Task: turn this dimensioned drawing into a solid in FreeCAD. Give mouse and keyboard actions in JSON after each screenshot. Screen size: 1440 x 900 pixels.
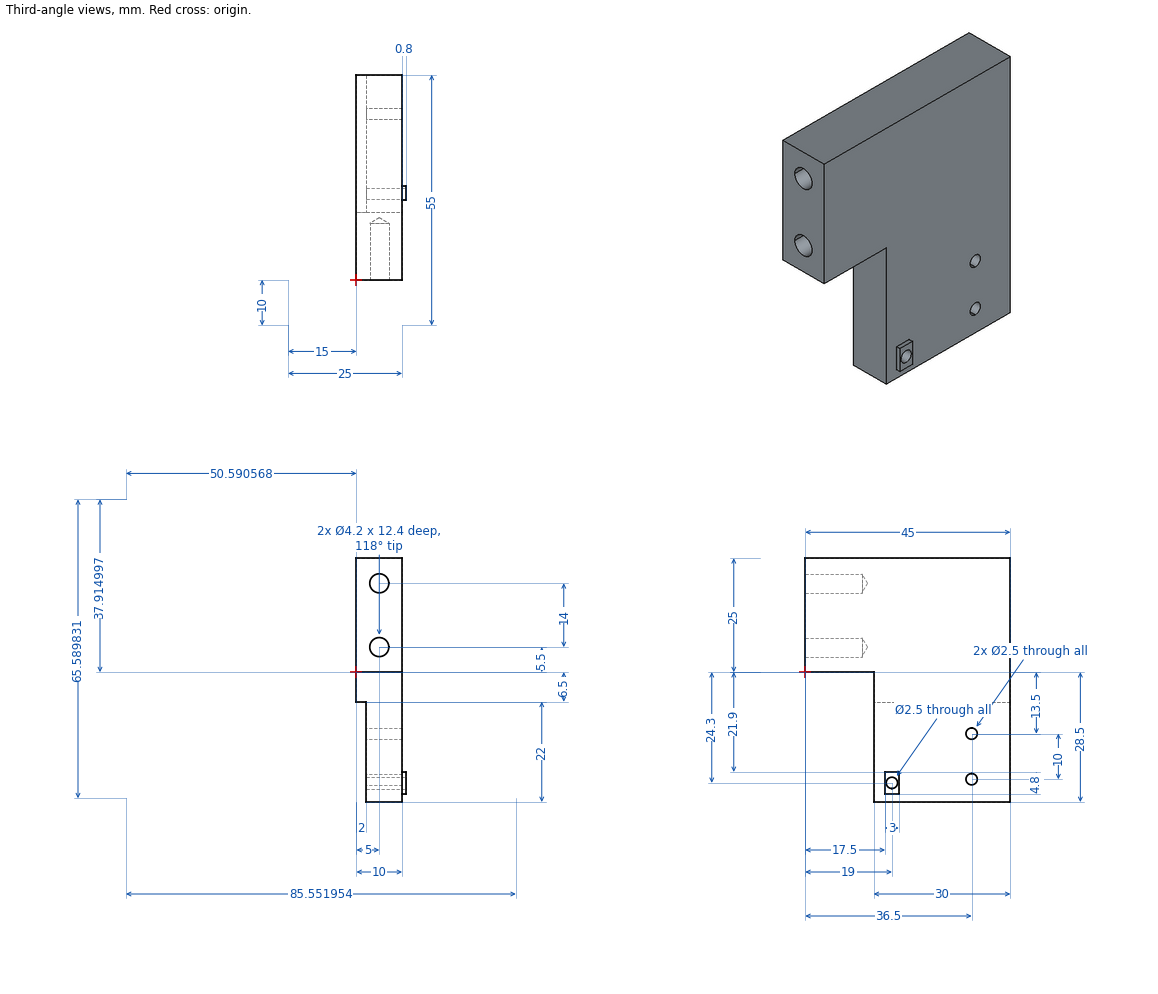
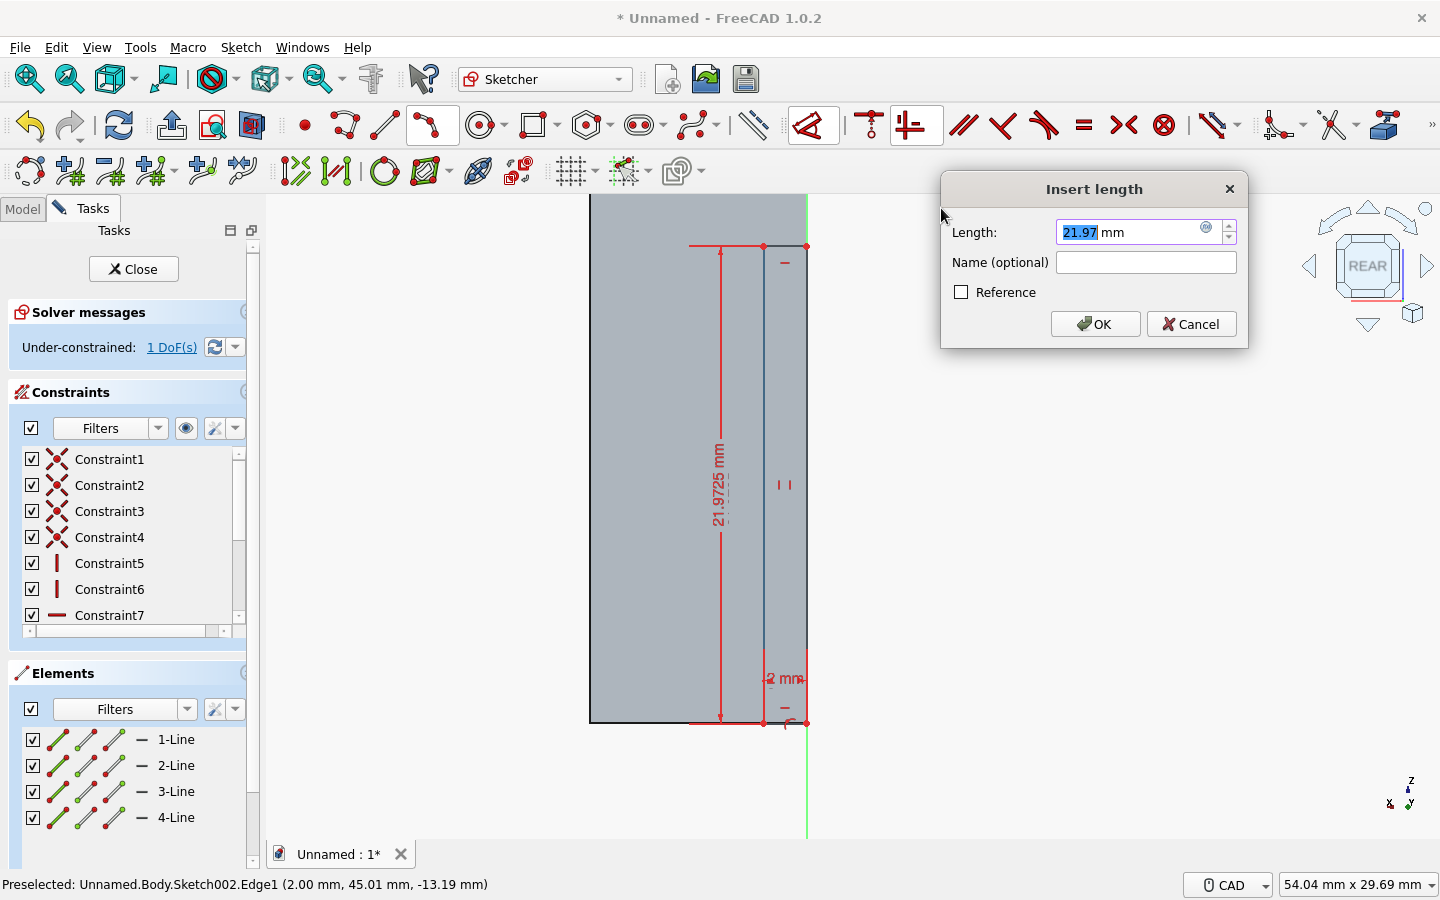
{"action": "type", "text": "22"}
{"action": "key", "text": "Return"}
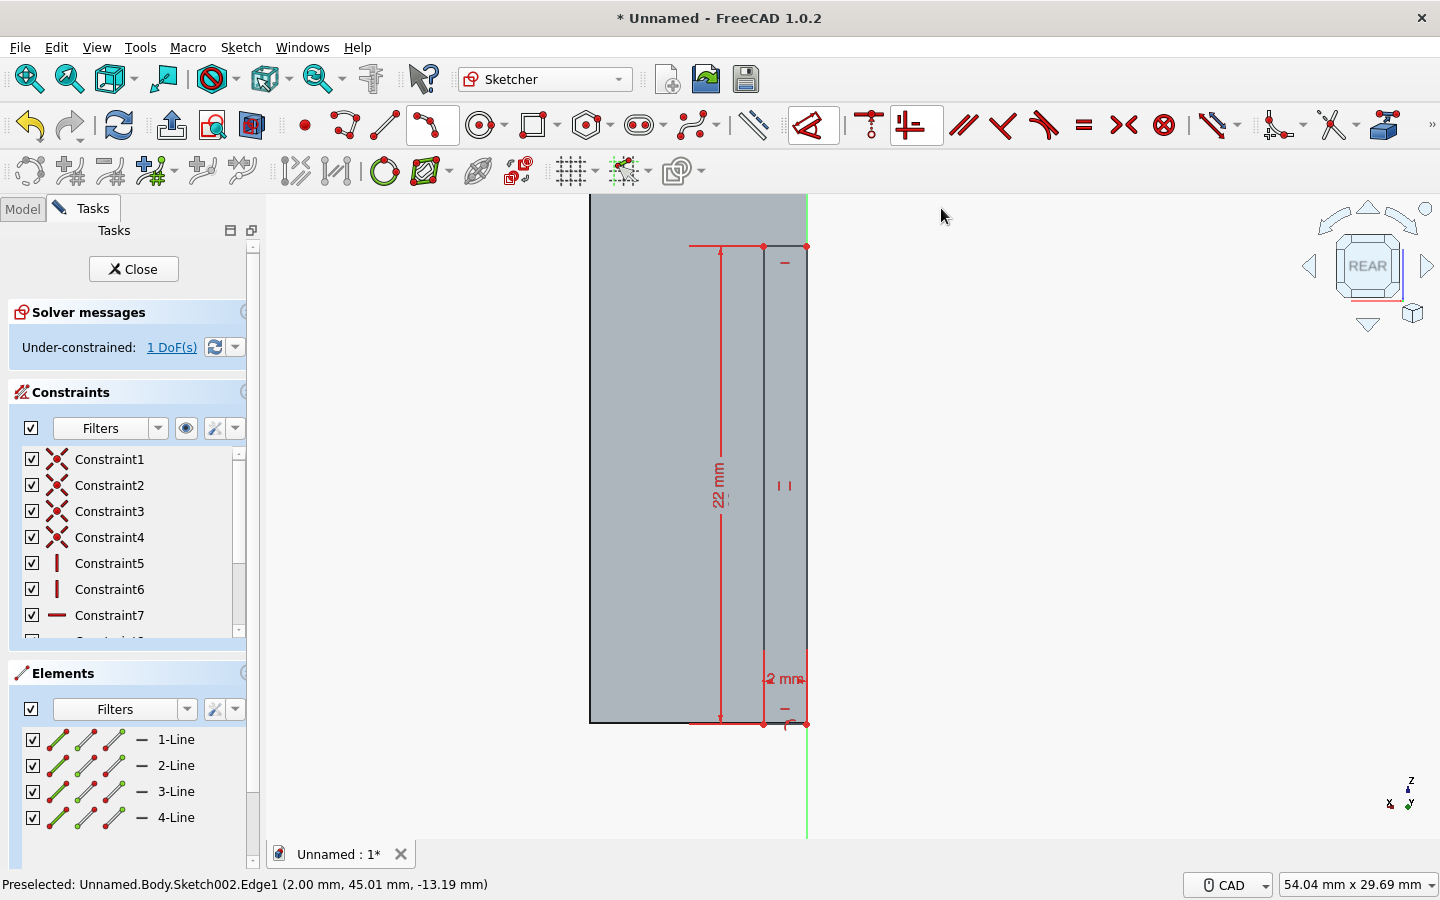
{"action": "left_click", "coordinate": [764, 246]}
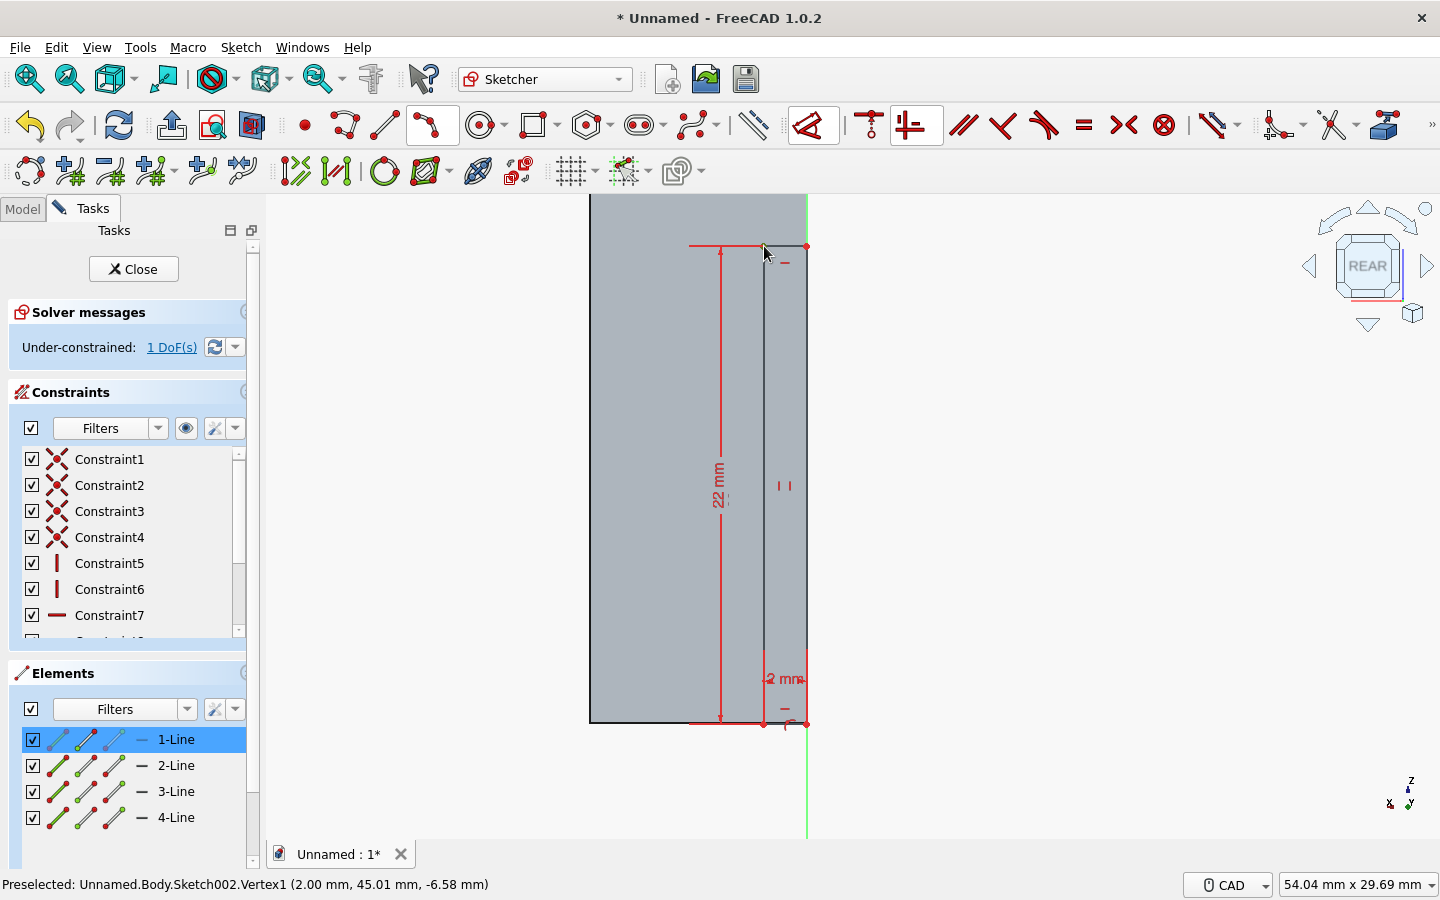
{"action": "left_click", "coordinate": [834, 126]}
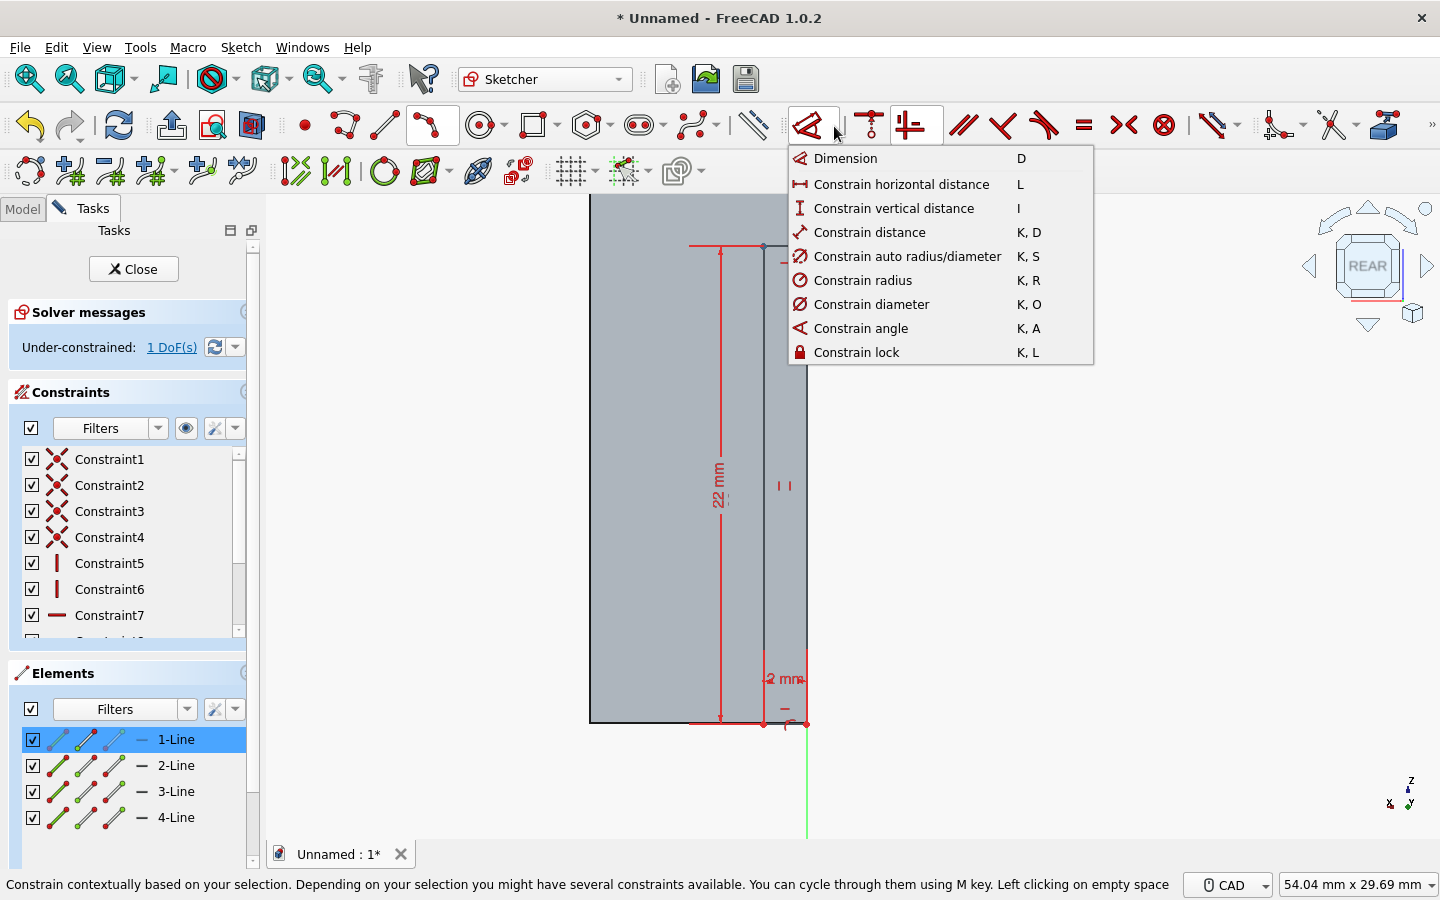
{"action": "left_click", "coordinate": [941, 208]}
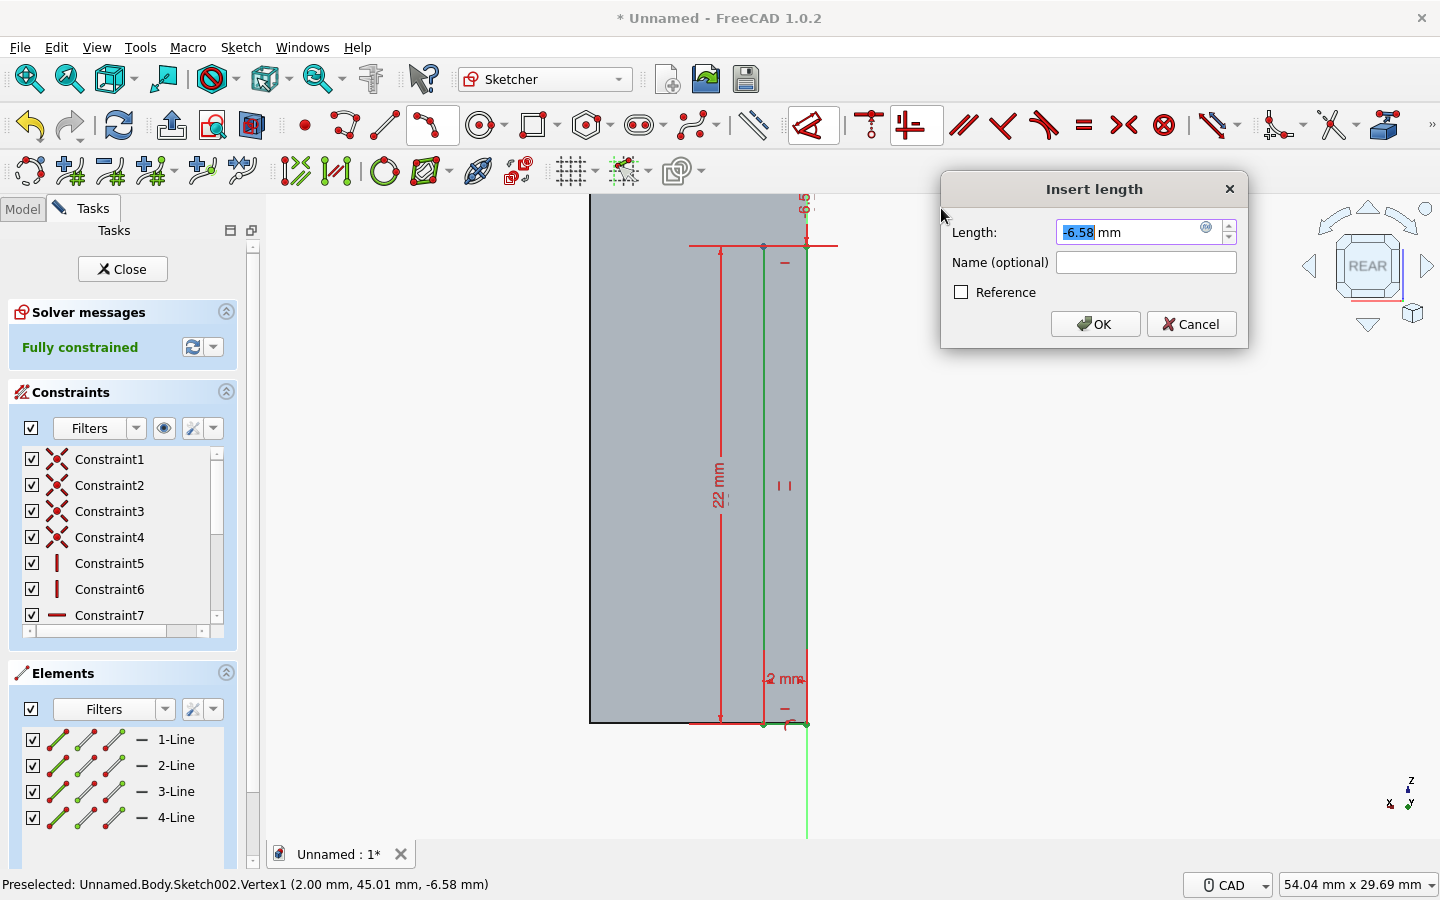
{"action": "type", "text": "-6.5"}
{"action": "key", "text": "Return"}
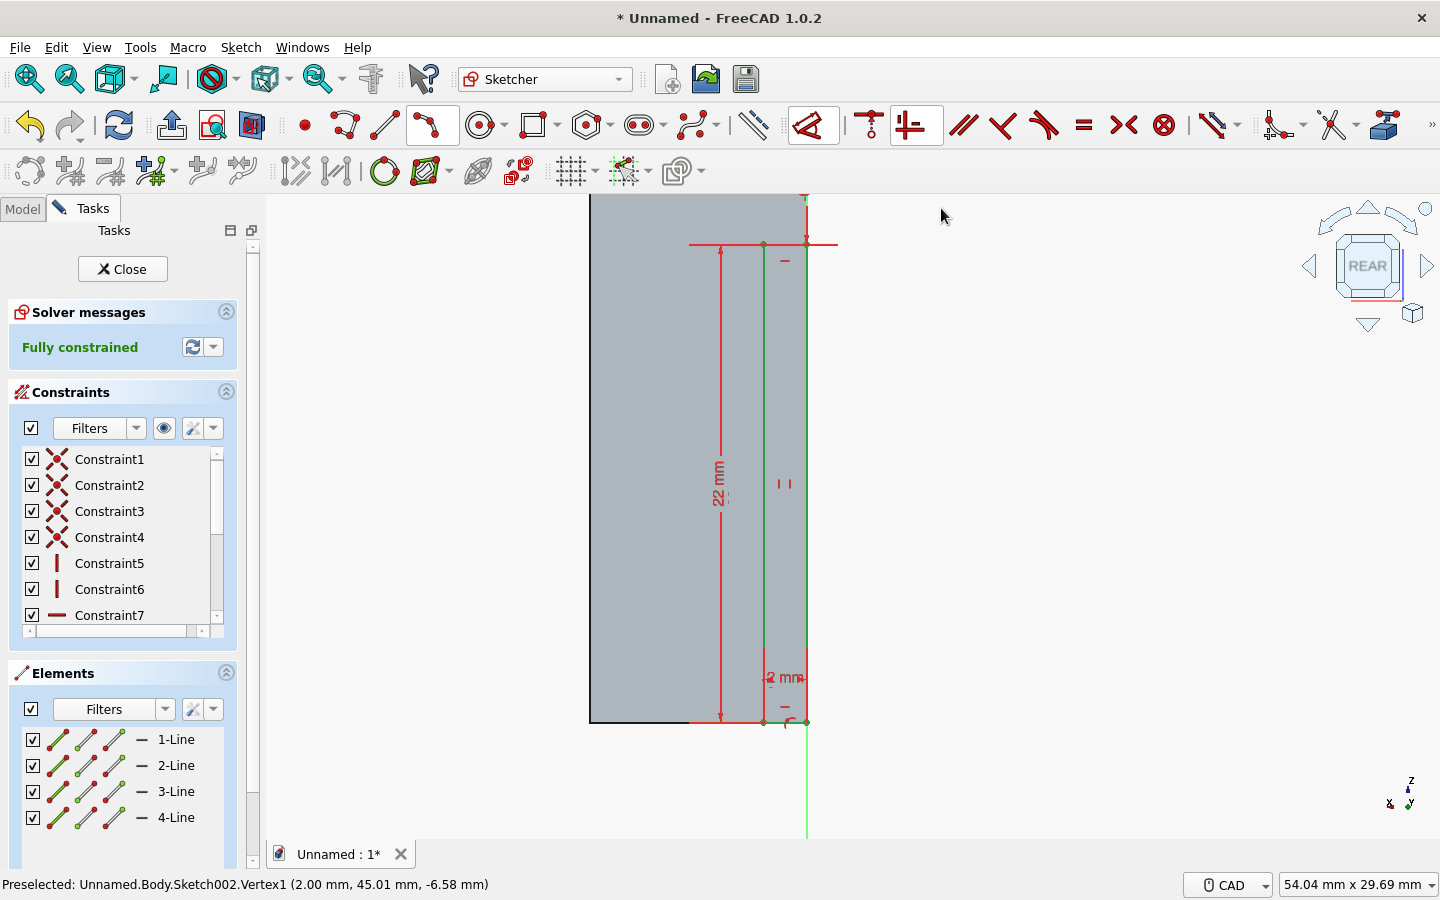
{"action": "left_click", "coordinate": [123, 269]}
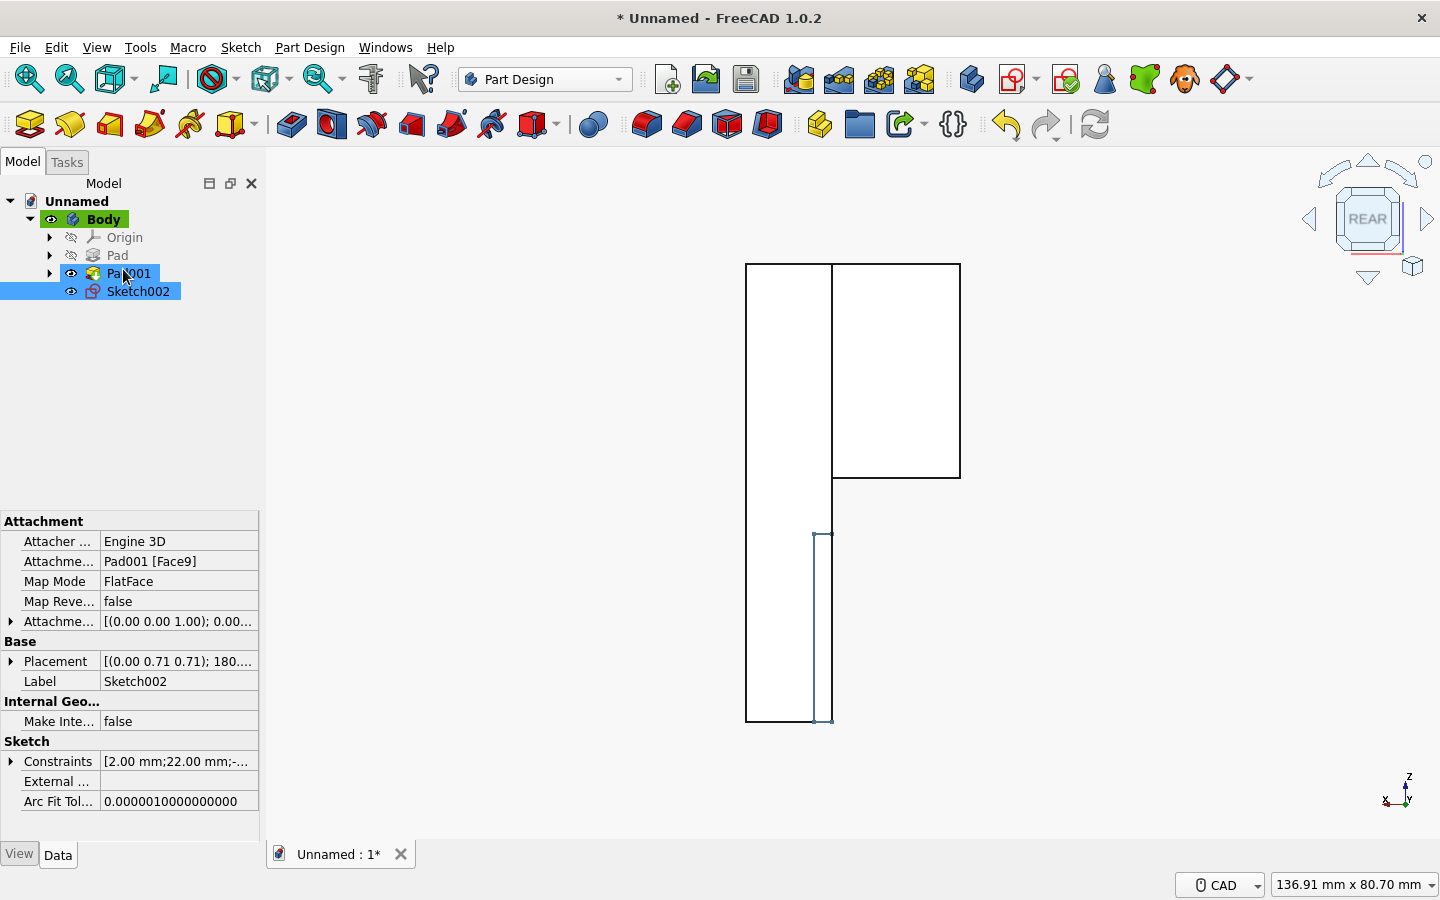
{"action": "left_click", "coordinate": [292, 124]}